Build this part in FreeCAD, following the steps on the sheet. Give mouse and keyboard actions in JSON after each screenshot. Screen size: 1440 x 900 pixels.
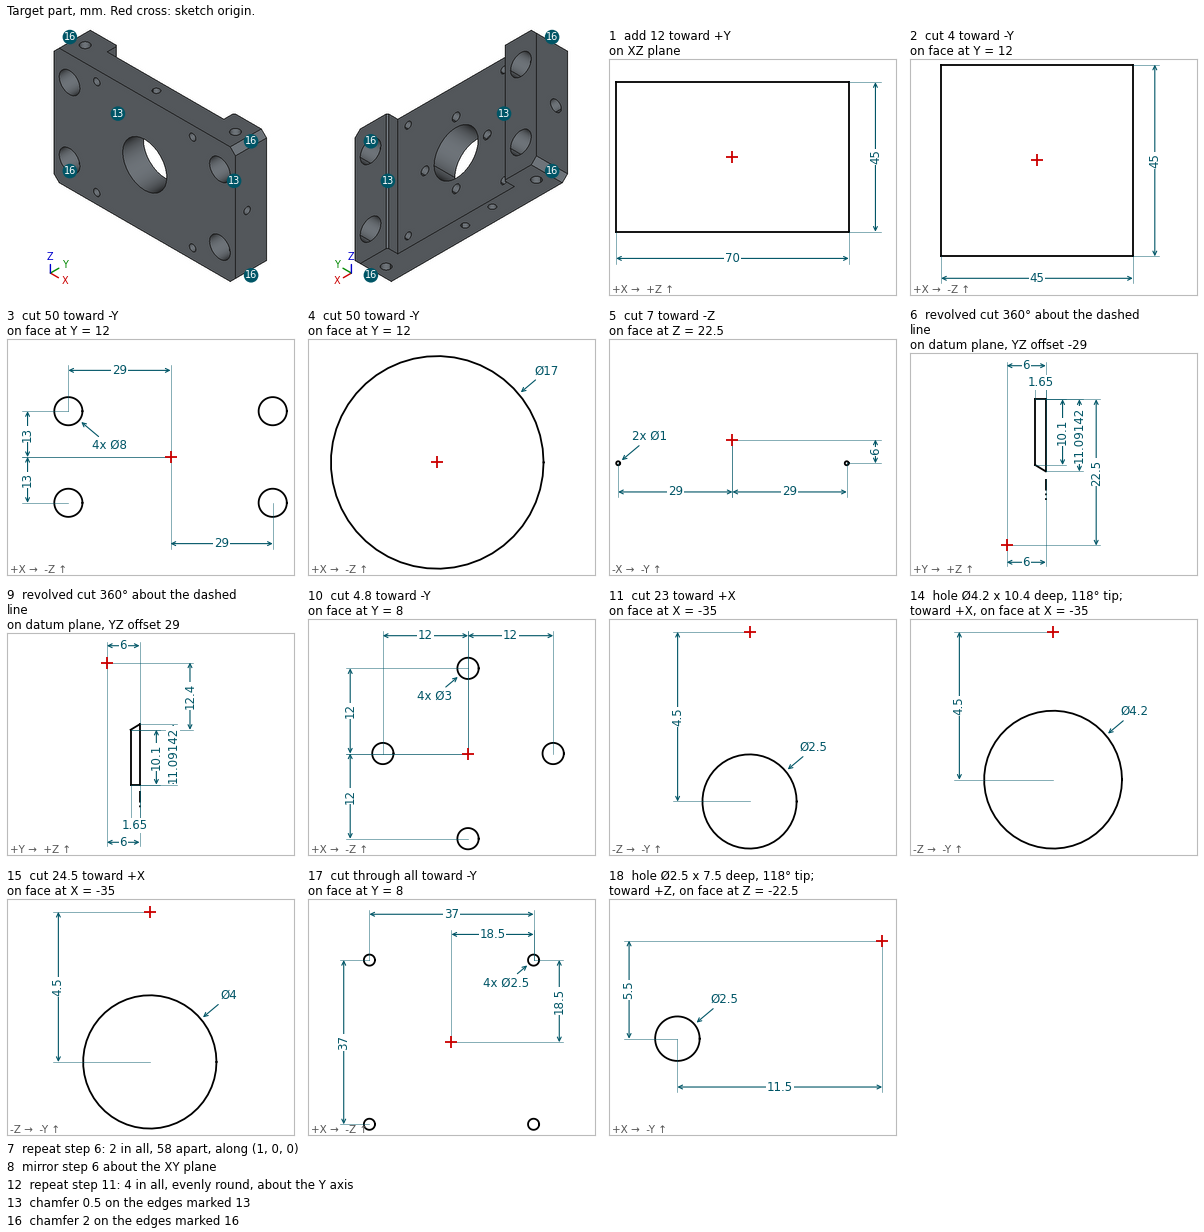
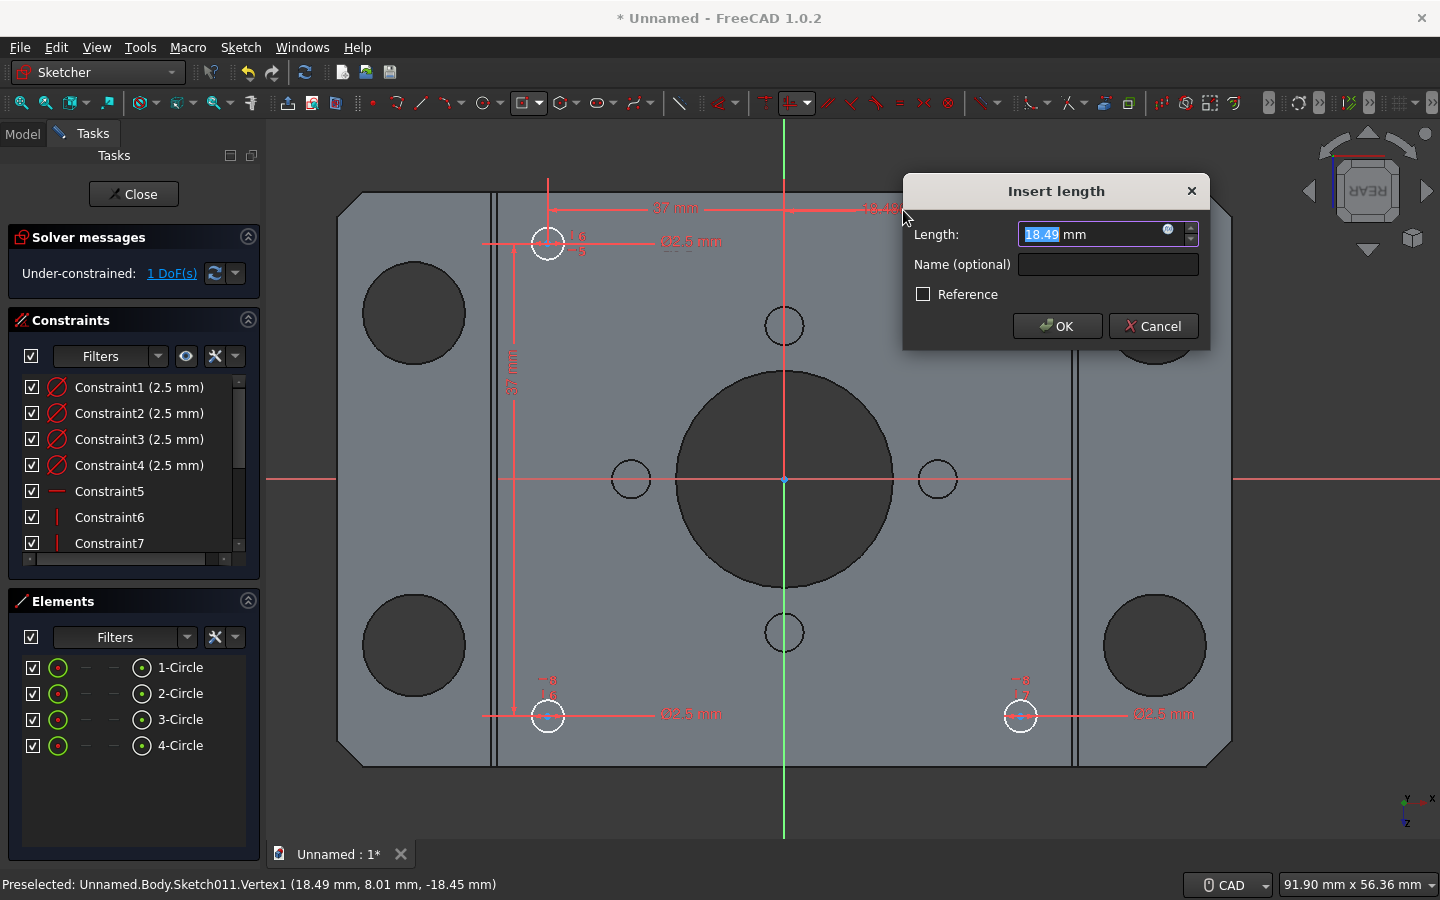
{"action": "type", "text": "18.5"}
{"action": "key", "text": "Return"}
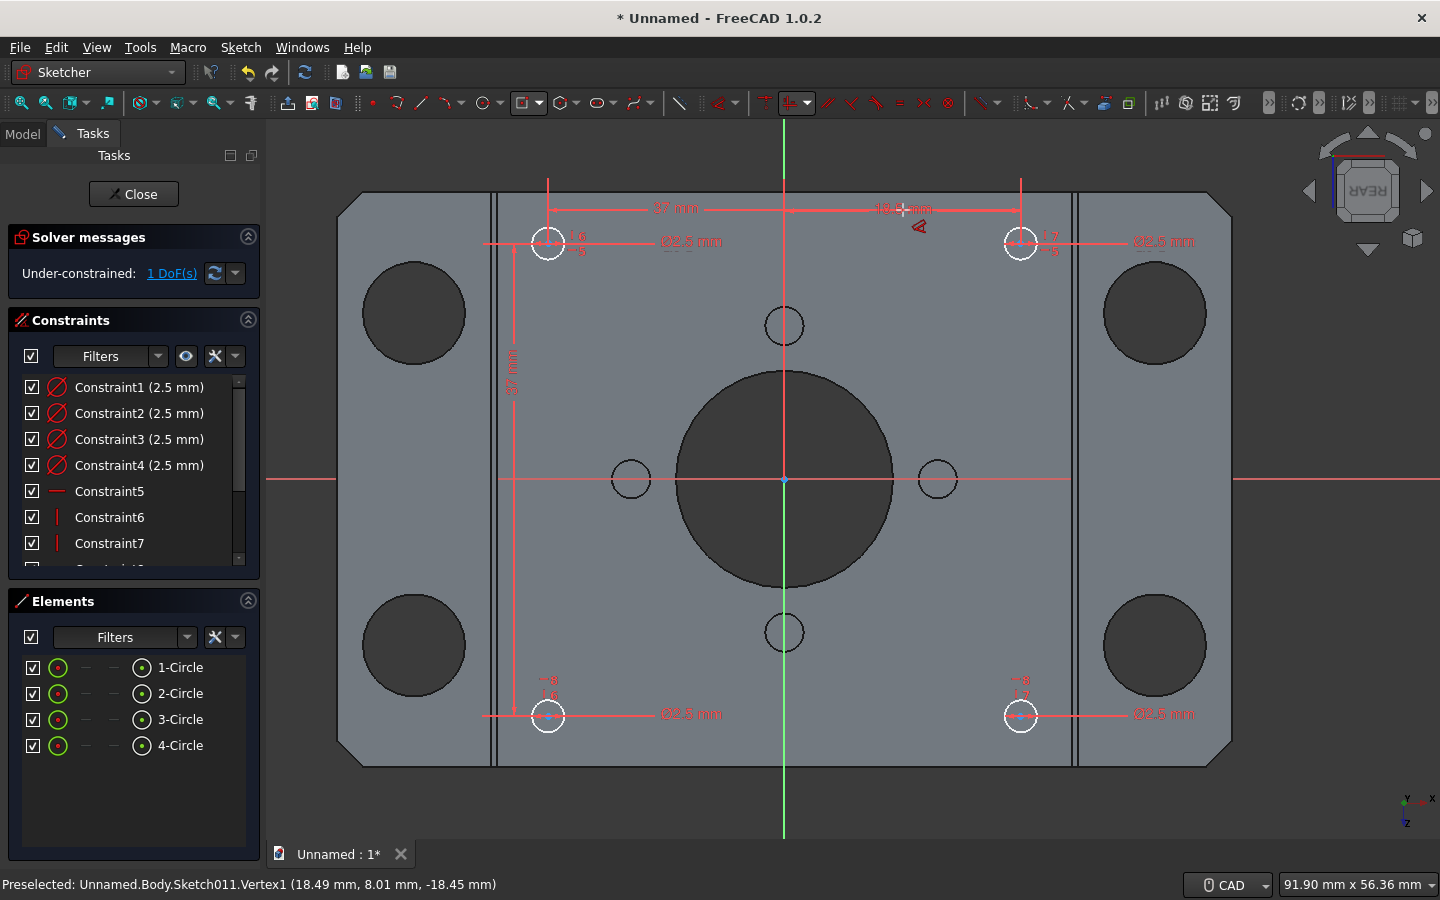
{"action": "left_click", "coordinate": [1021, 244]}
{"action": "left_click", "coordinate": [1055, 361]}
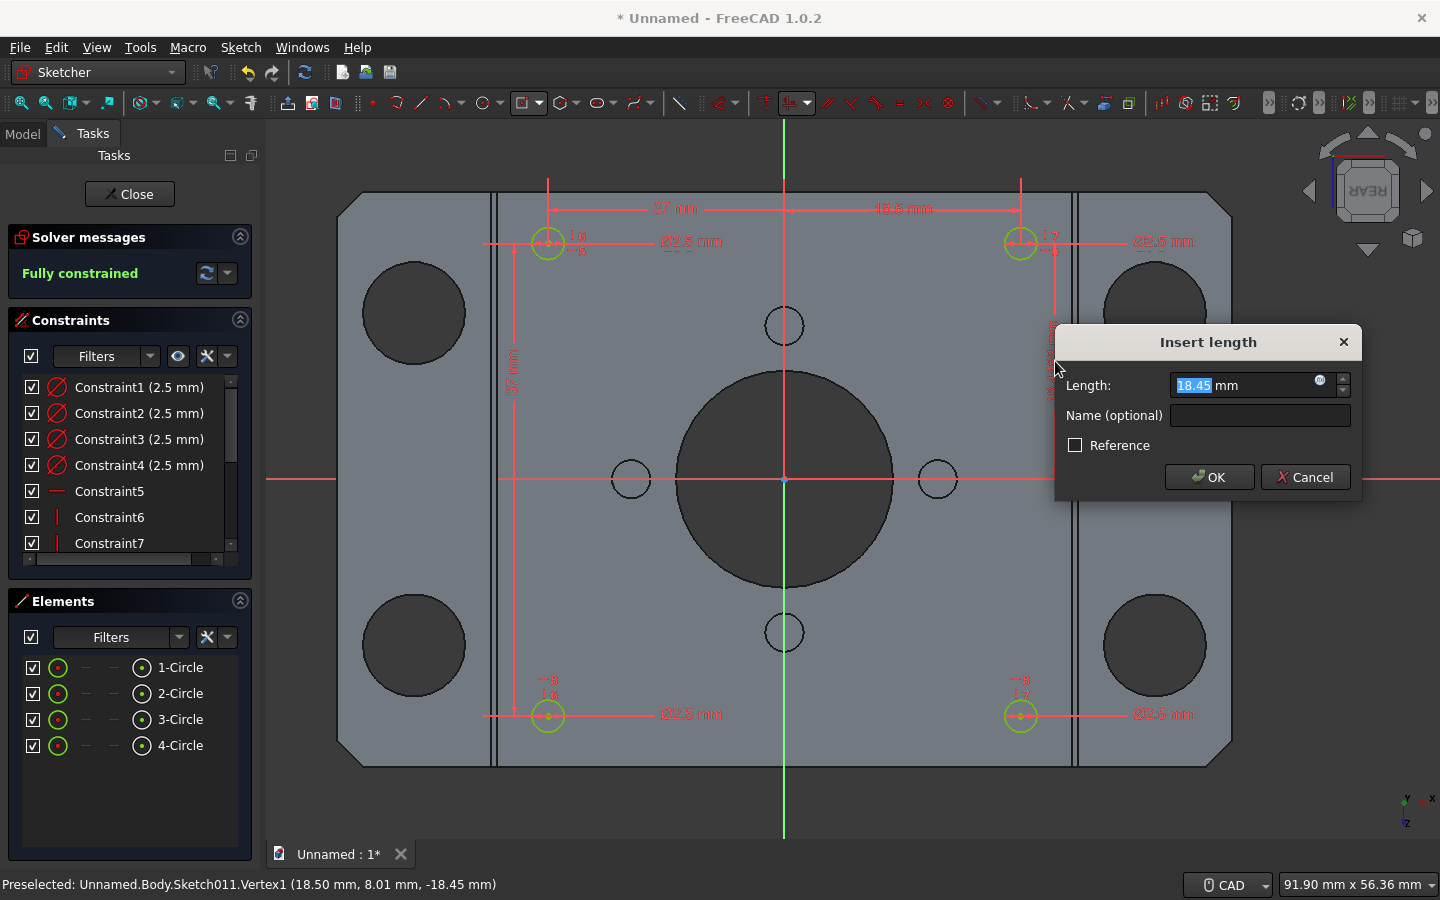
{"action": "type", "text": "18.5"}
{"action": "key", "text": "Return"}
{"action": "key", "text": "Escape"}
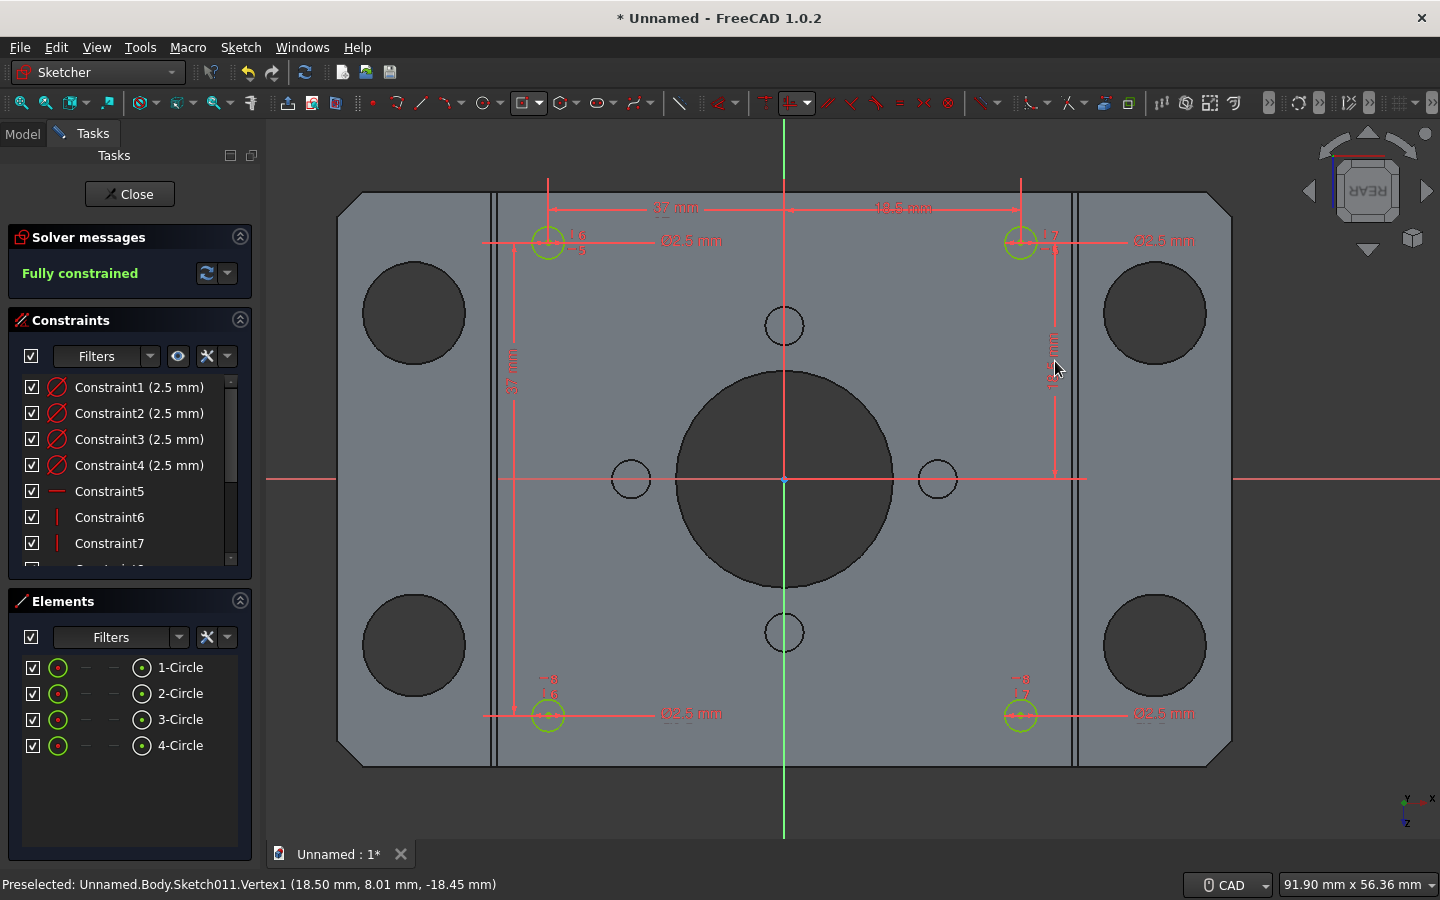
{"action": "left_click", "coordinate": [130, 194]}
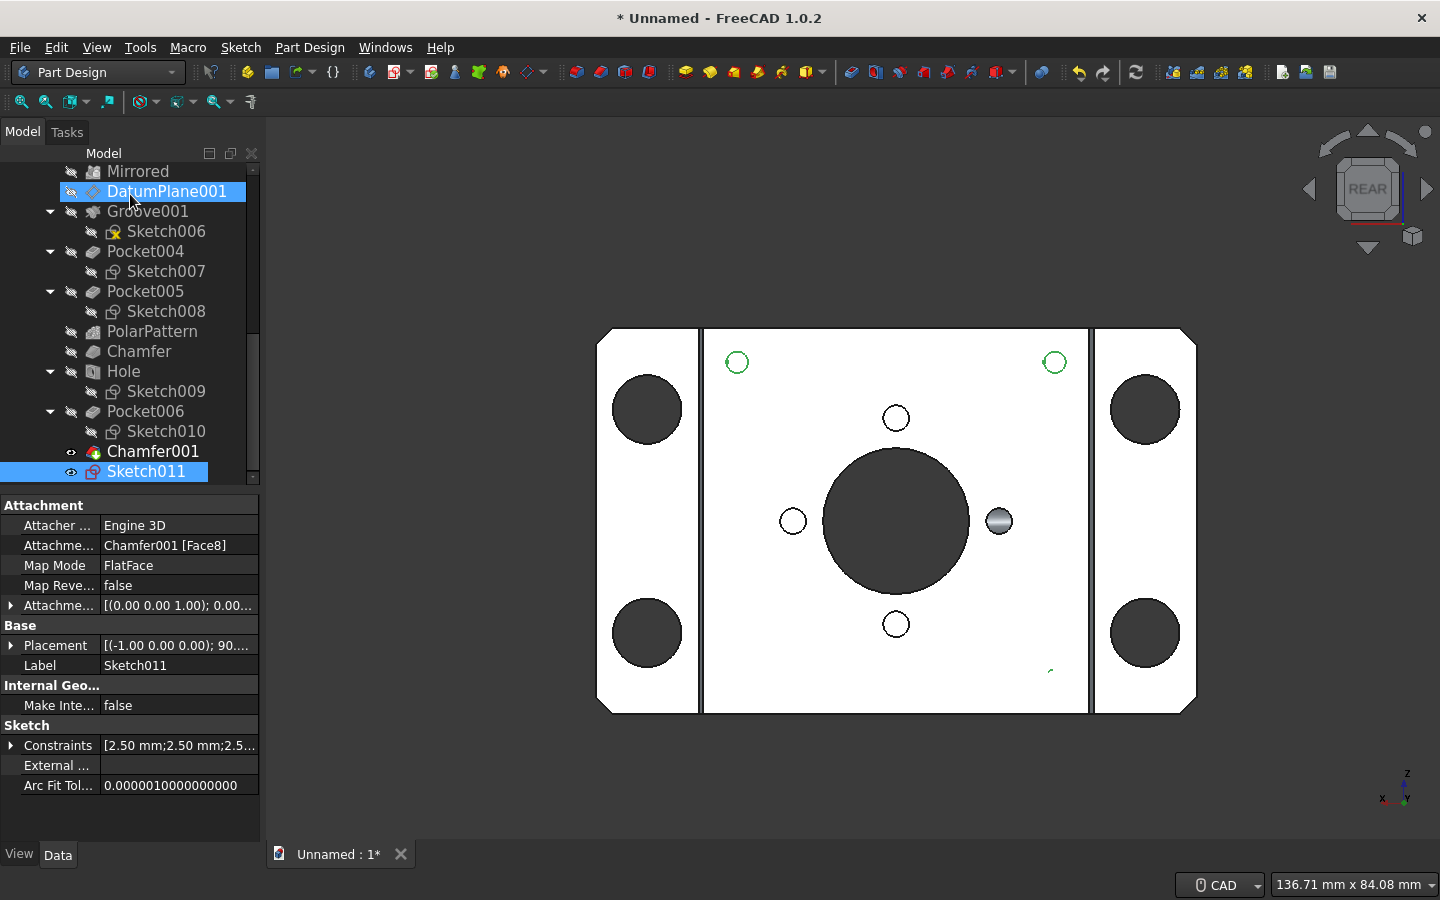
{"action": "left_click", "coordinate": [852, 72]}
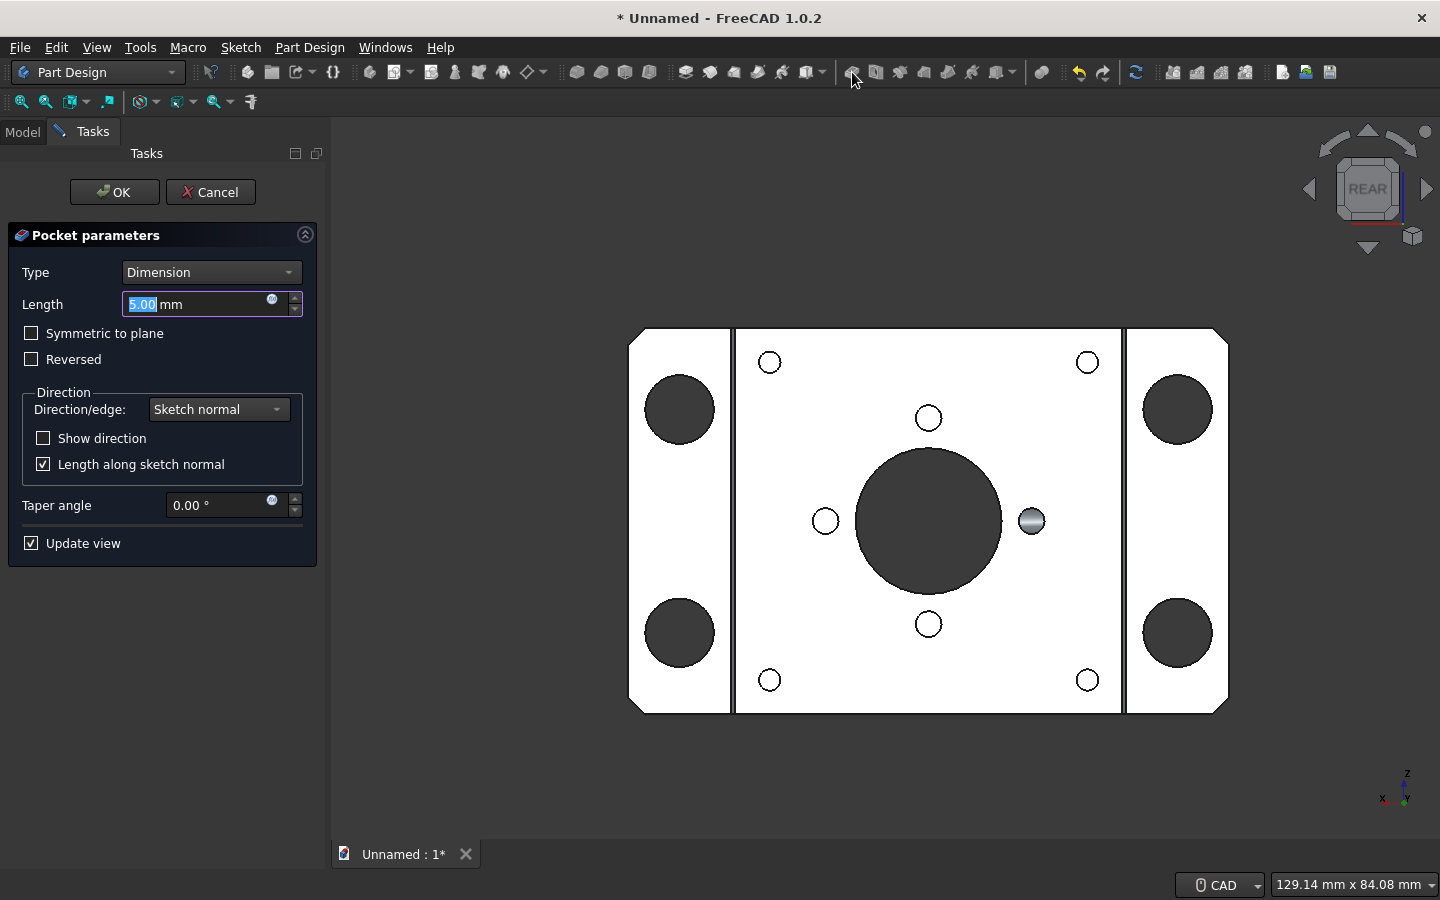
{"action": "left_click", "coordinate": [212, 272]}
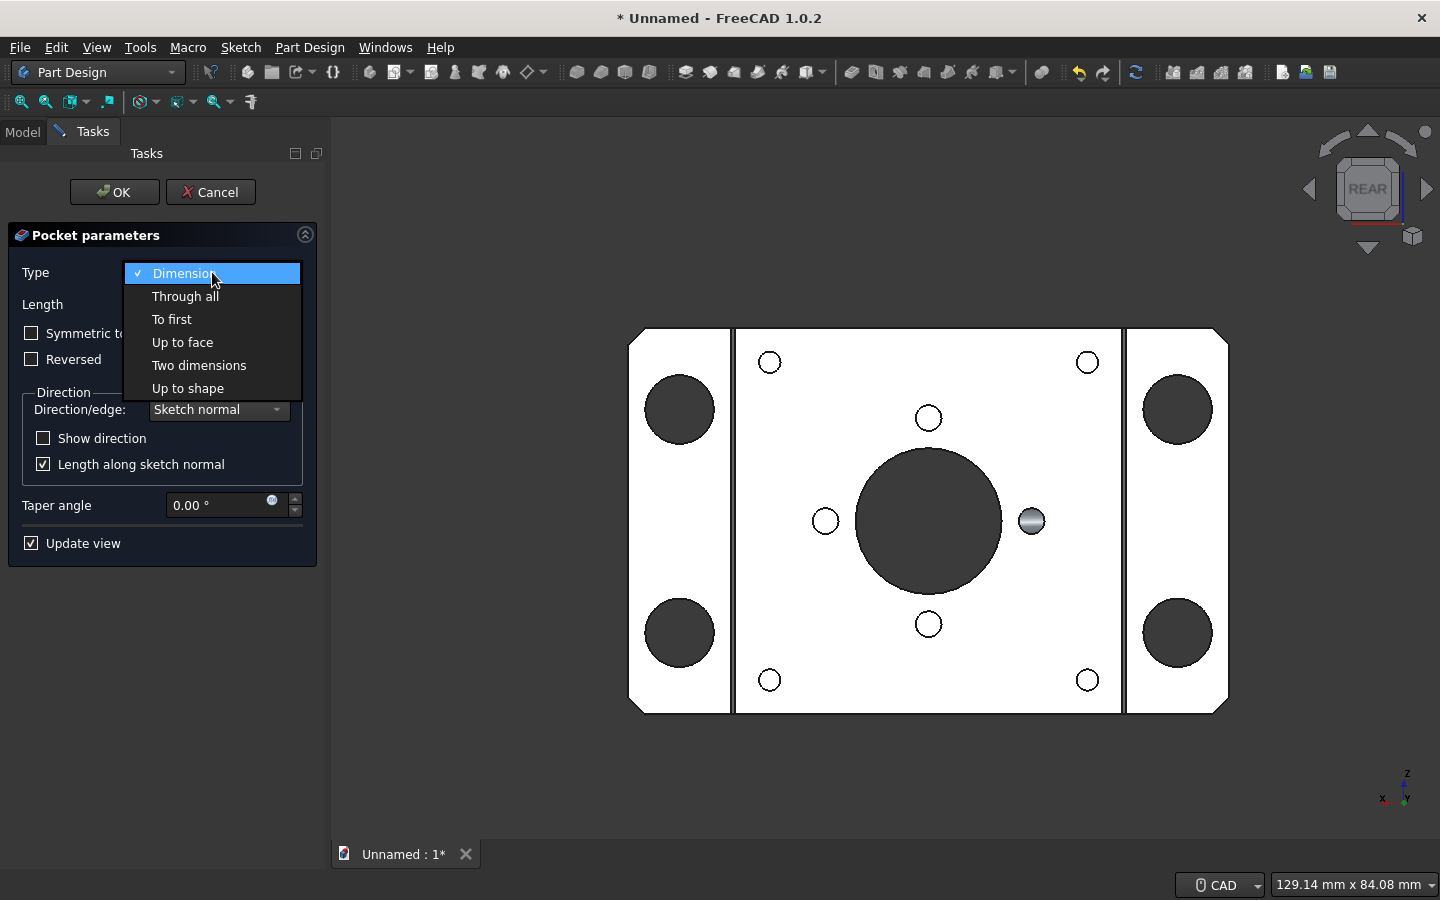
{"action": "left_click", "coordinate": [212, 296]}